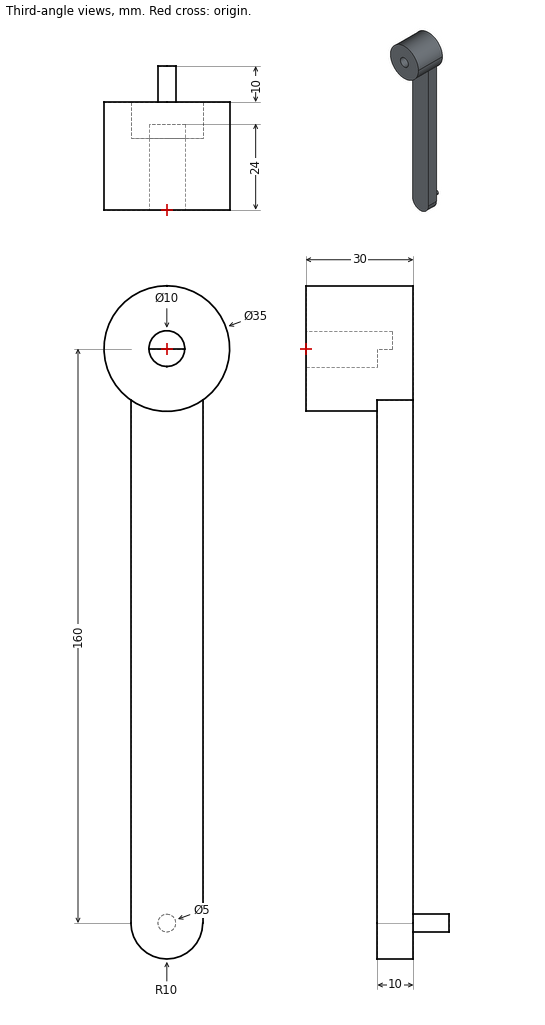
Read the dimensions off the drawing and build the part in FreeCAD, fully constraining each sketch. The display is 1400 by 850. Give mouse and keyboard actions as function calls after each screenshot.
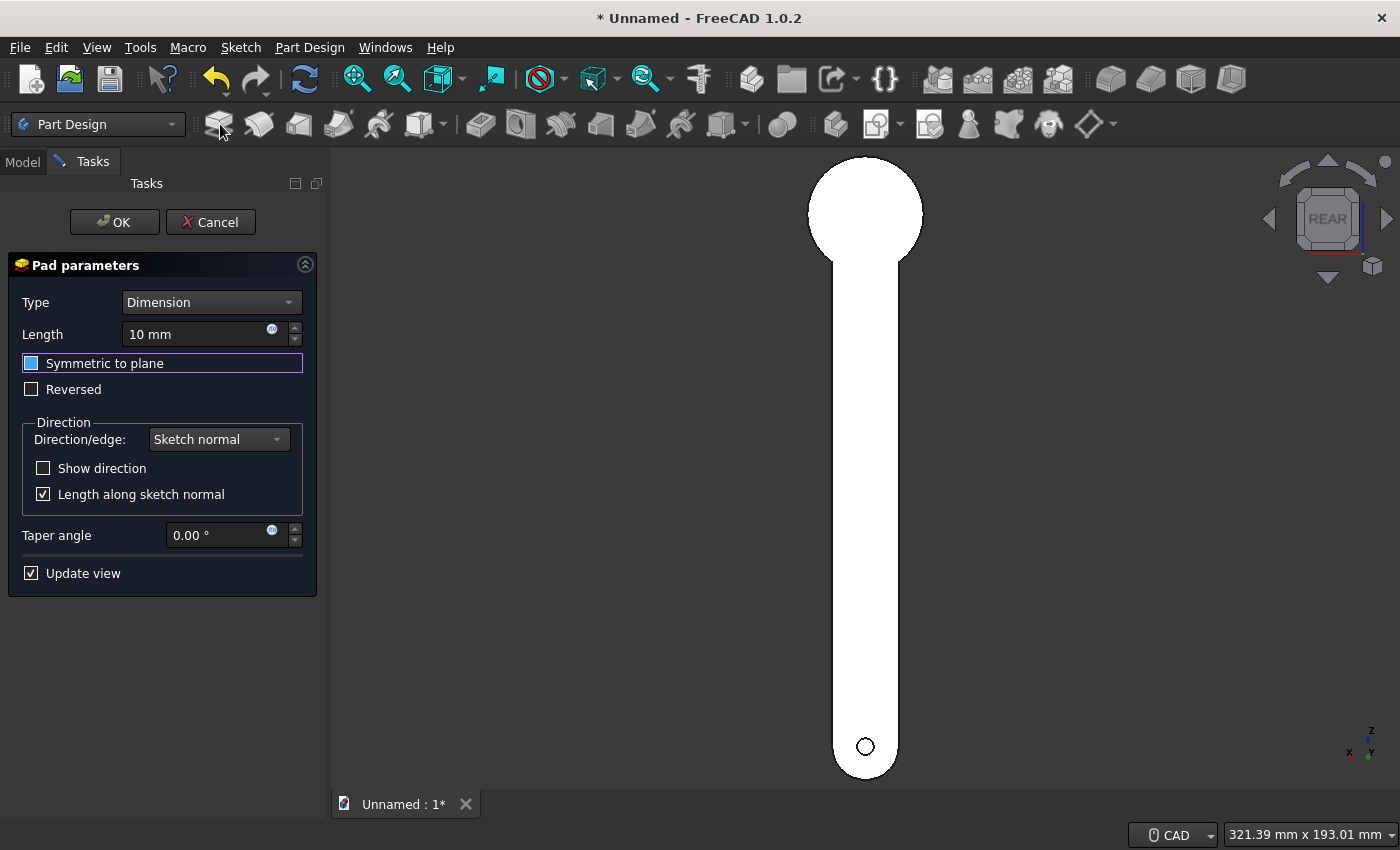
click(115, 222)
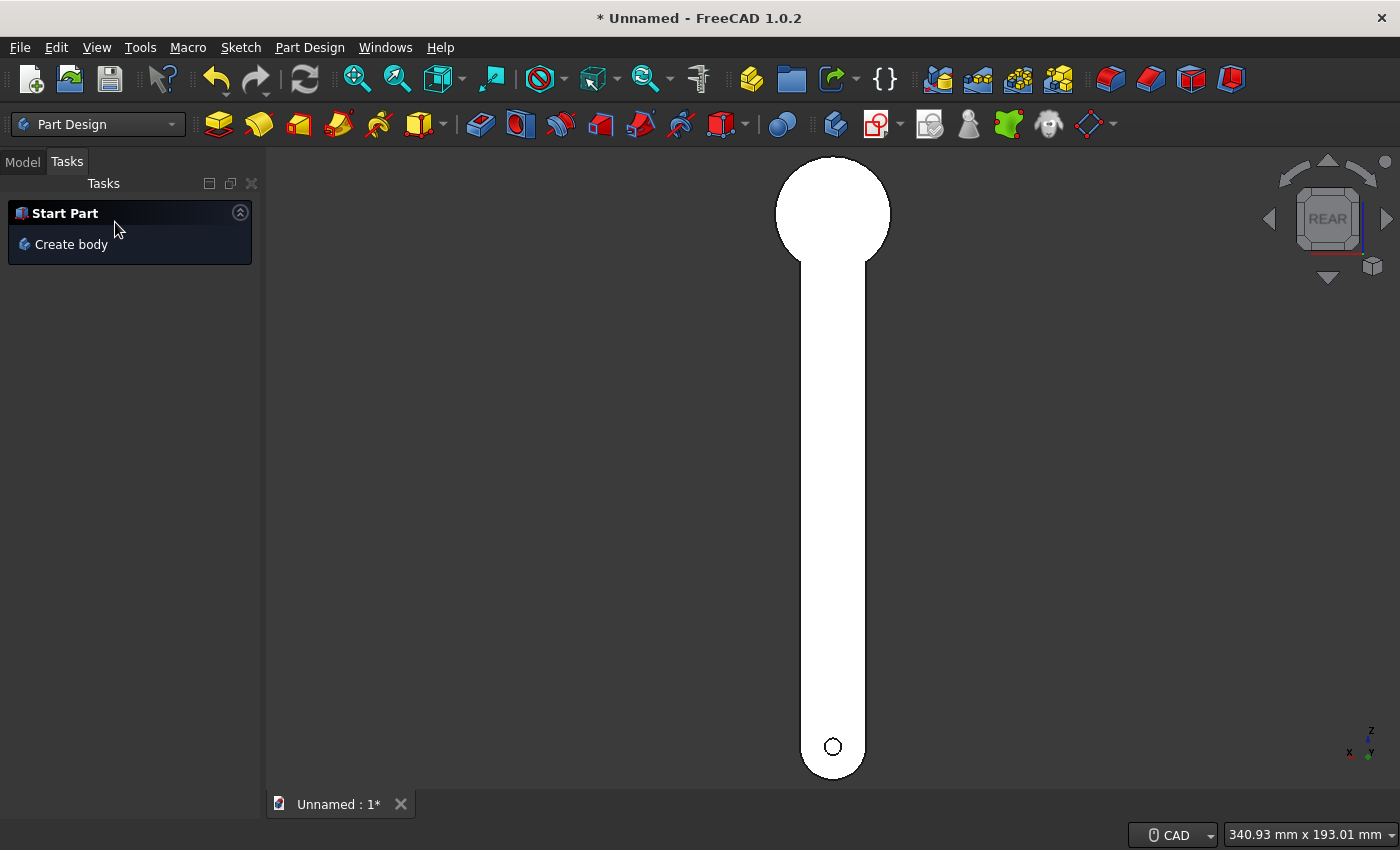
key(0)